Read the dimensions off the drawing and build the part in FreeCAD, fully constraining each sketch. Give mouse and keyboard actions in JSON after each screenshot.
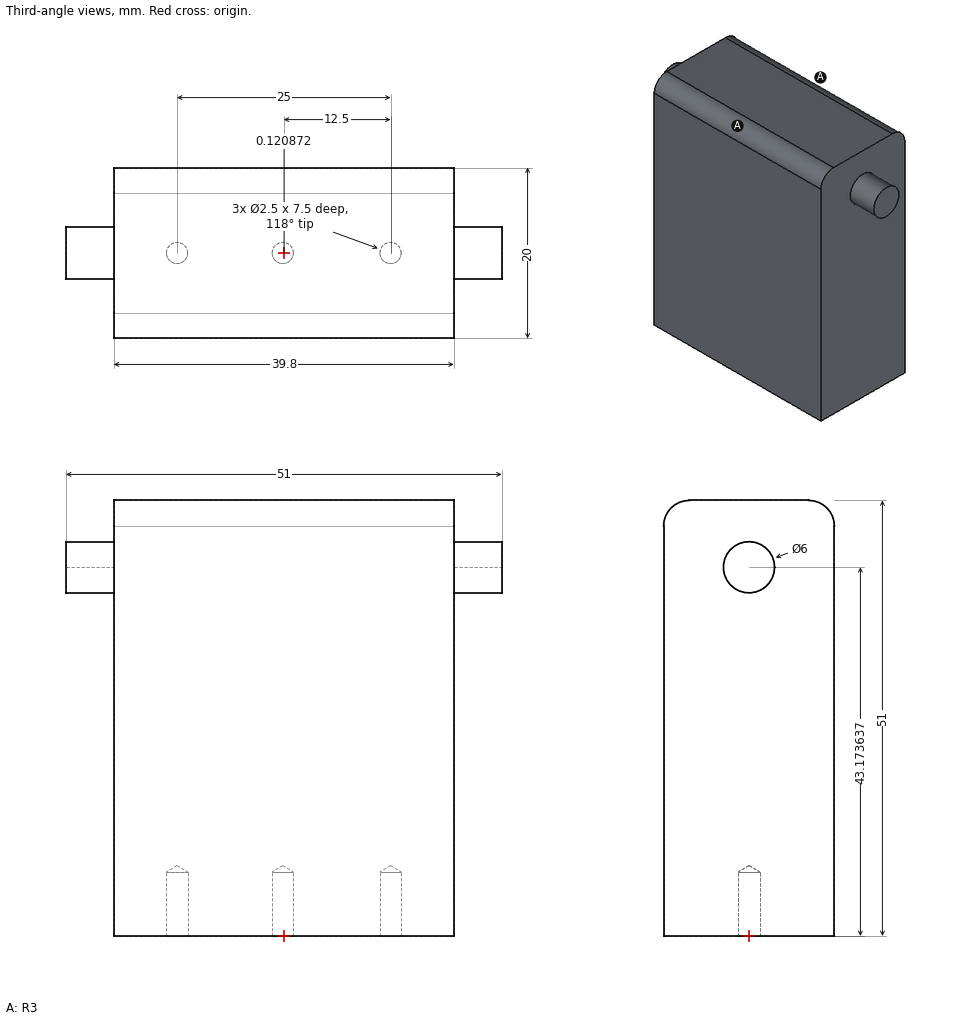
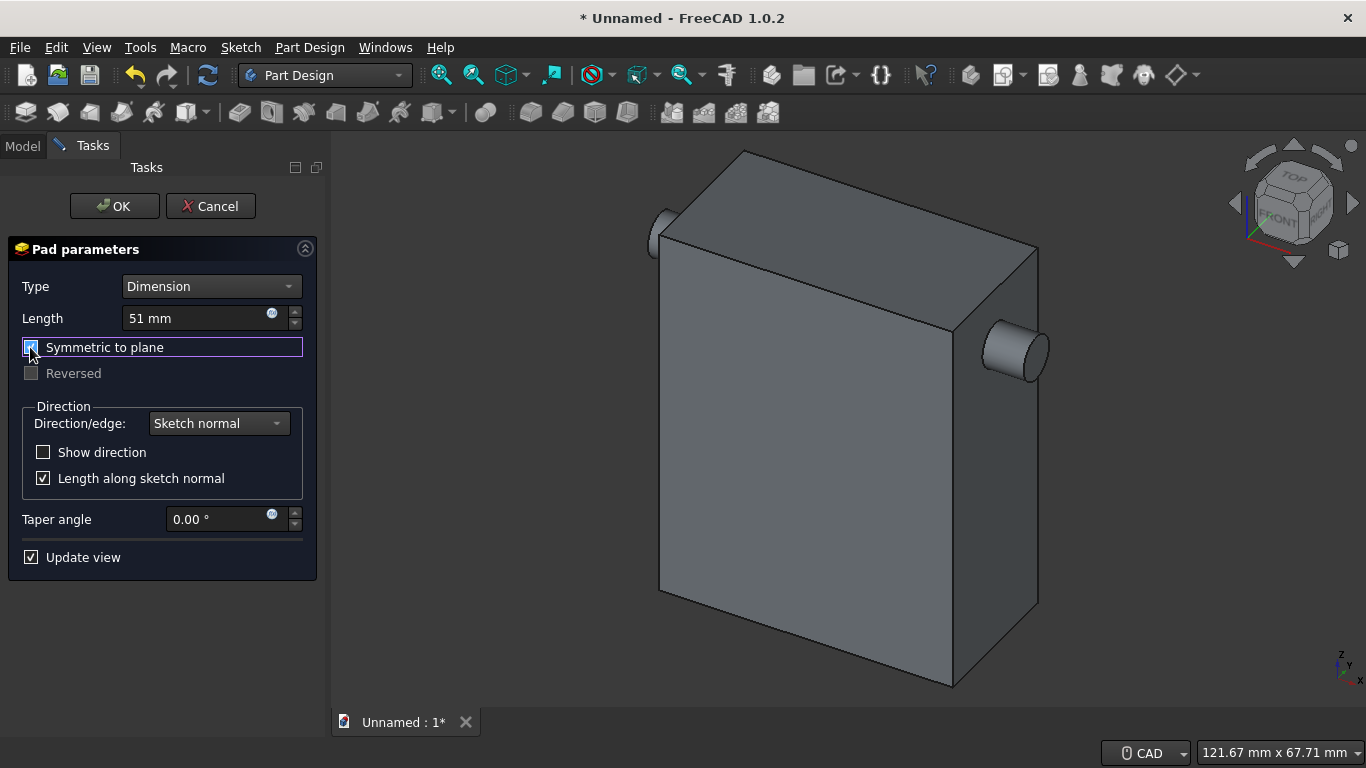
{"action": "left_click", "coordinate": [115, 206]}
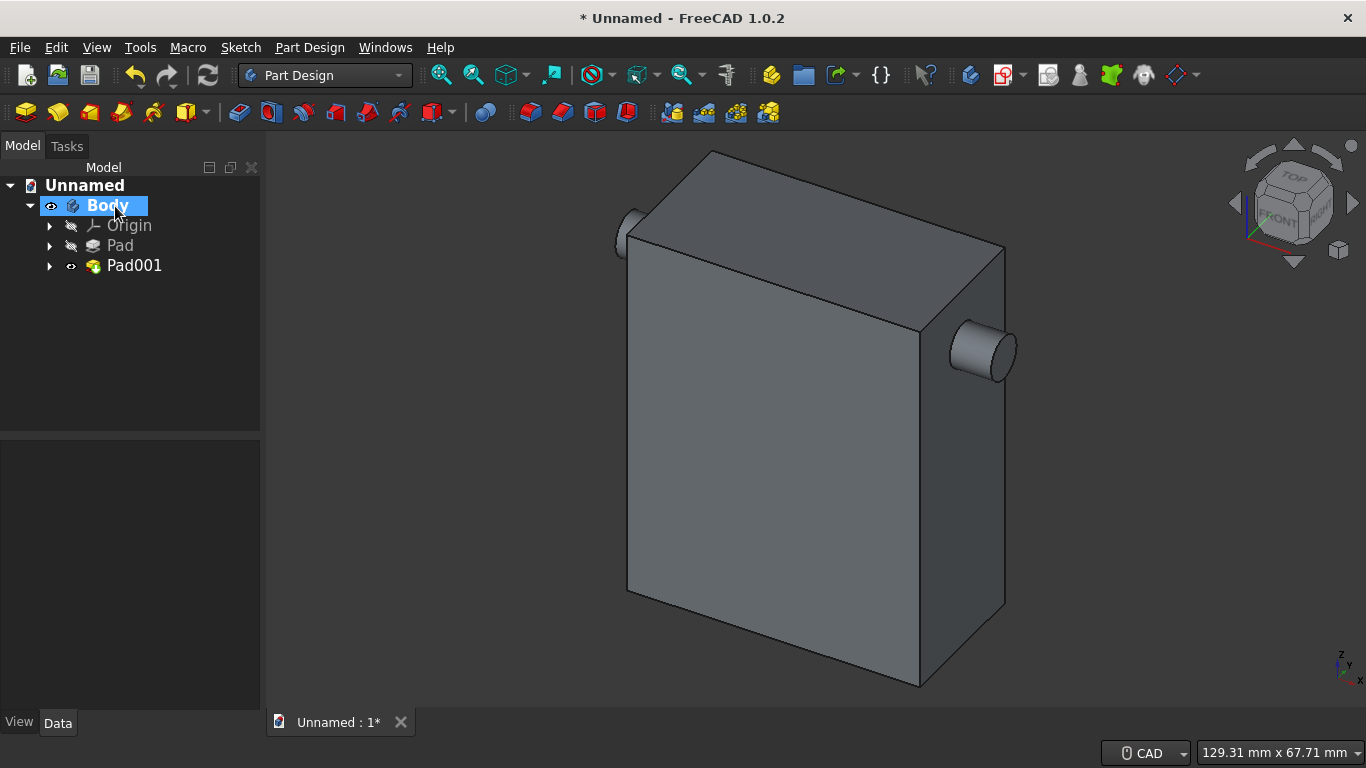
{"action": "key", "text": "5"}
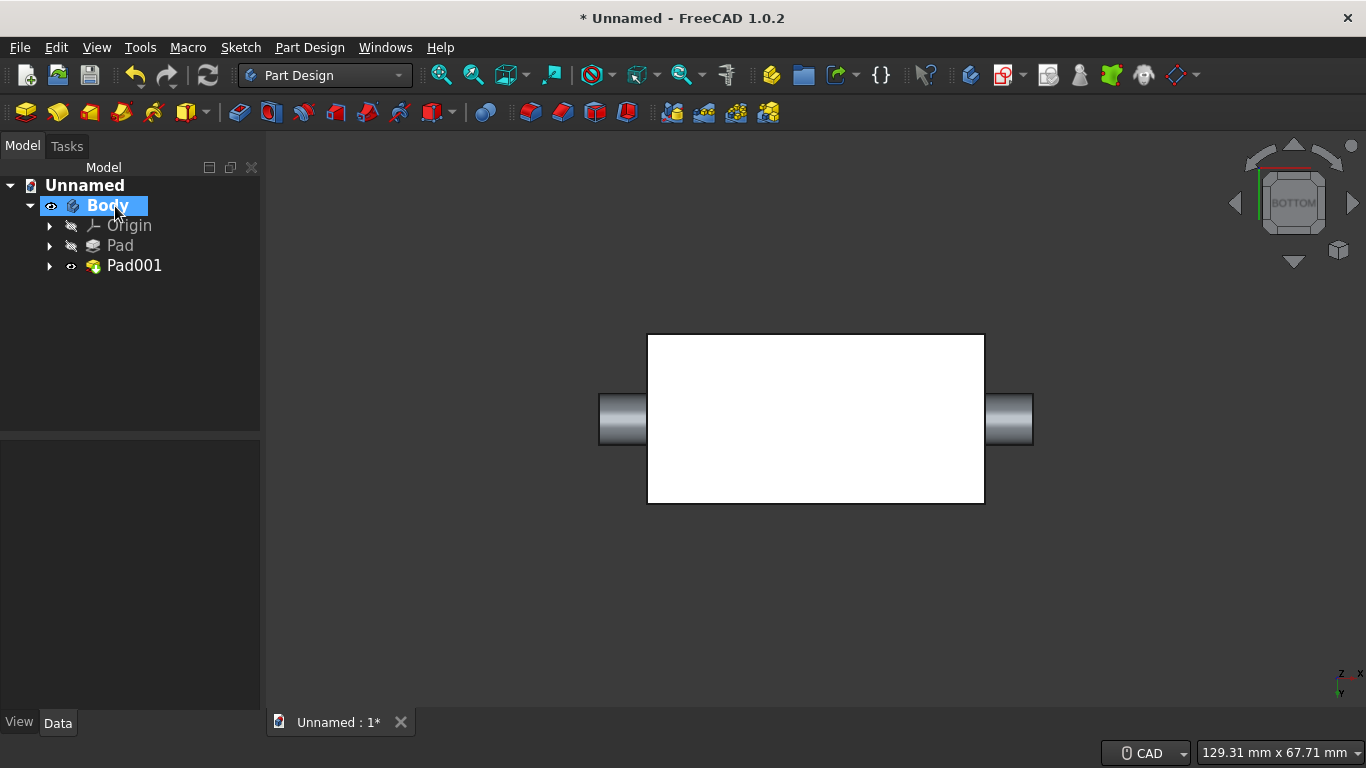
{"action": "key", "text": "v f"}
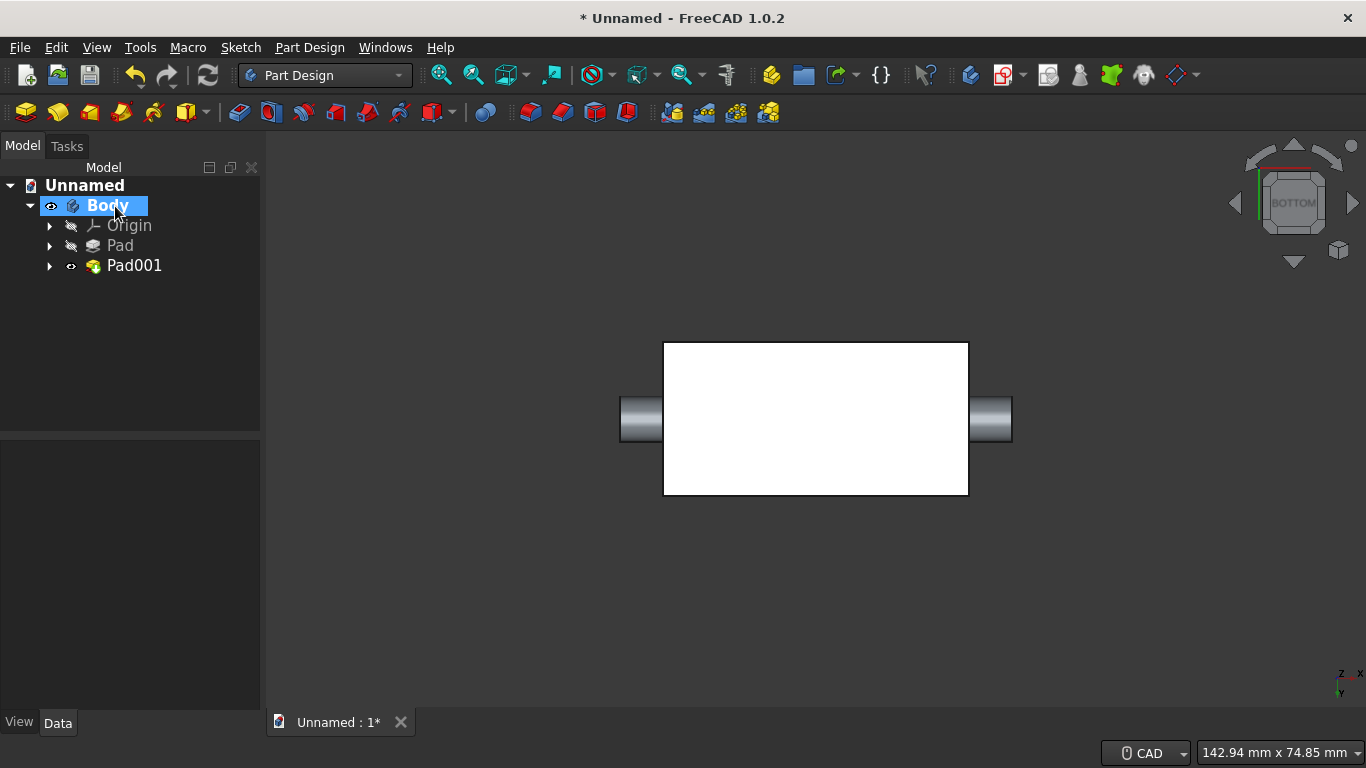
{"action": "left_click", "coordinate": [860, 418]}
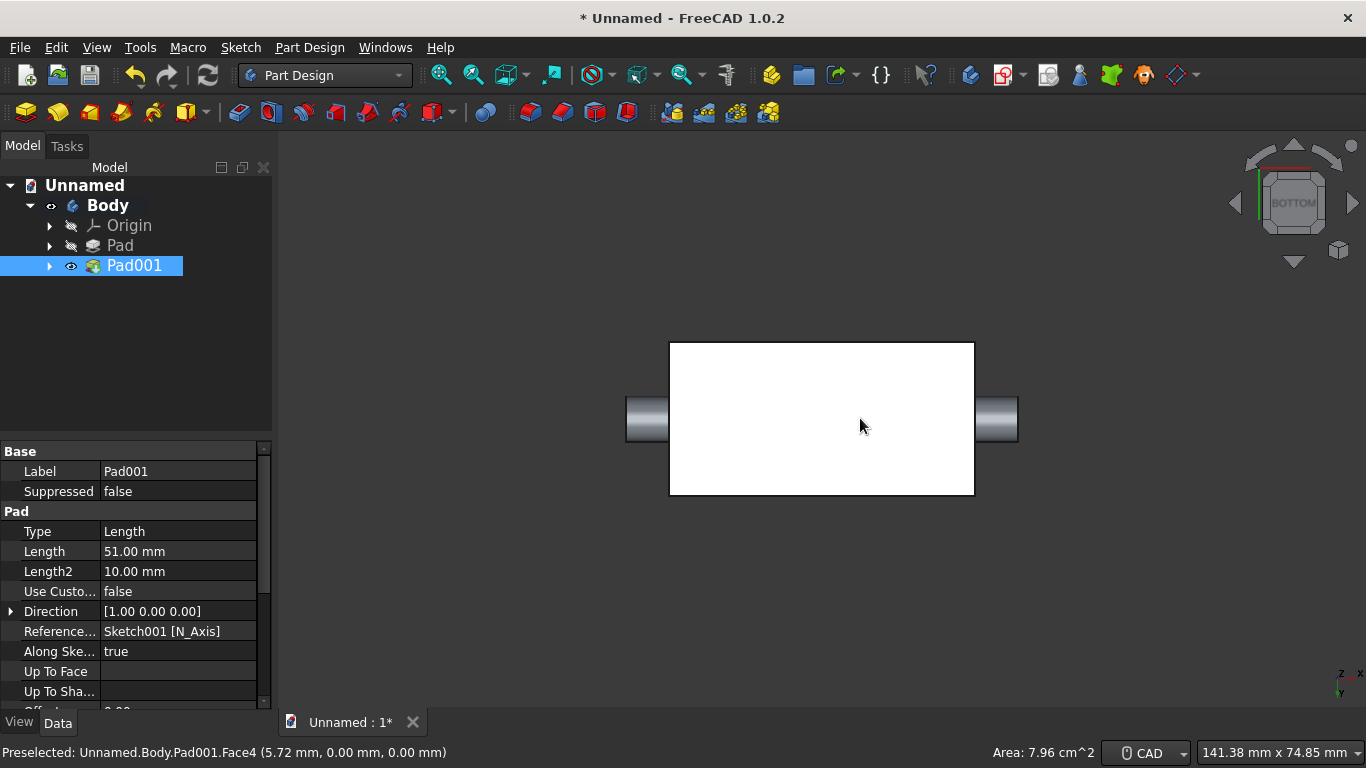
{"action": "left_click", "coordinate": [1004, 76]}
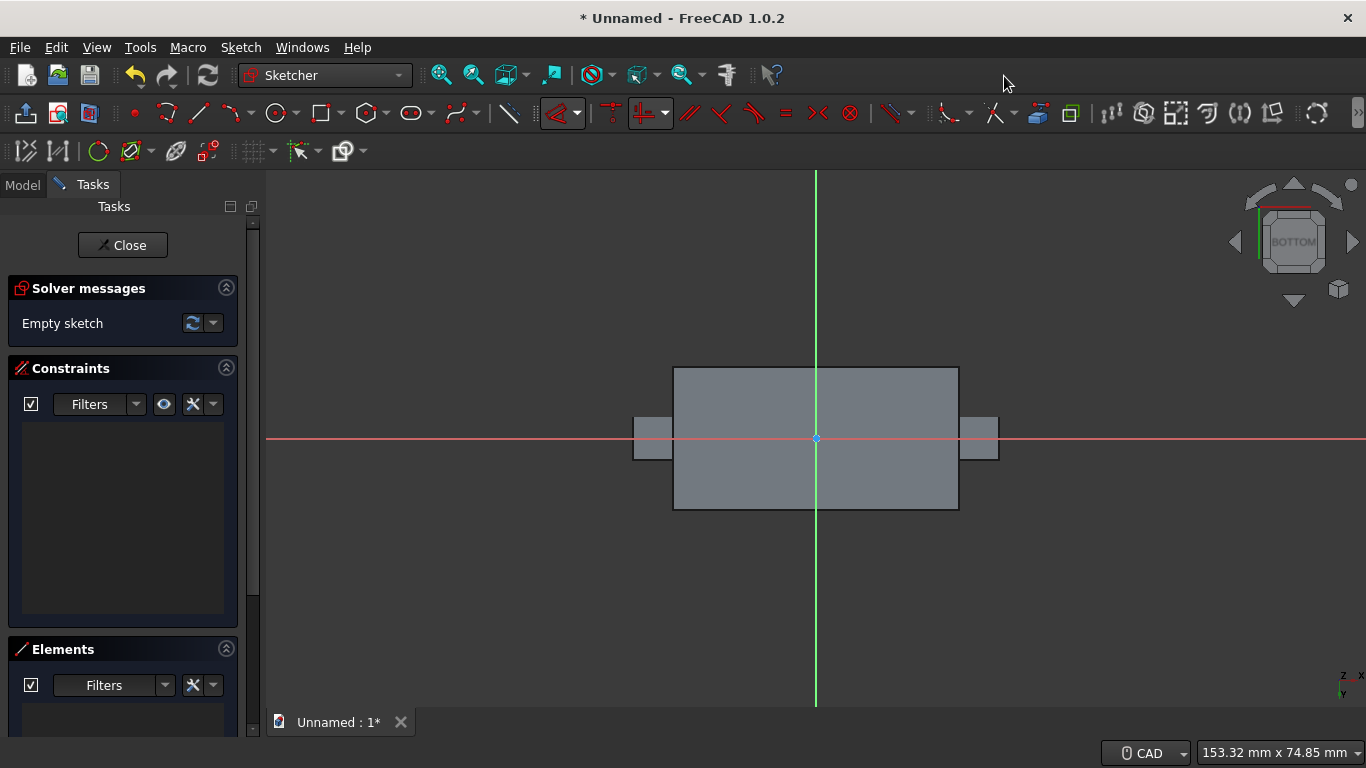
{"action": "scroll", "coordinate": [846, 438], "scroll_direction": "up", "scroll_amount": 6}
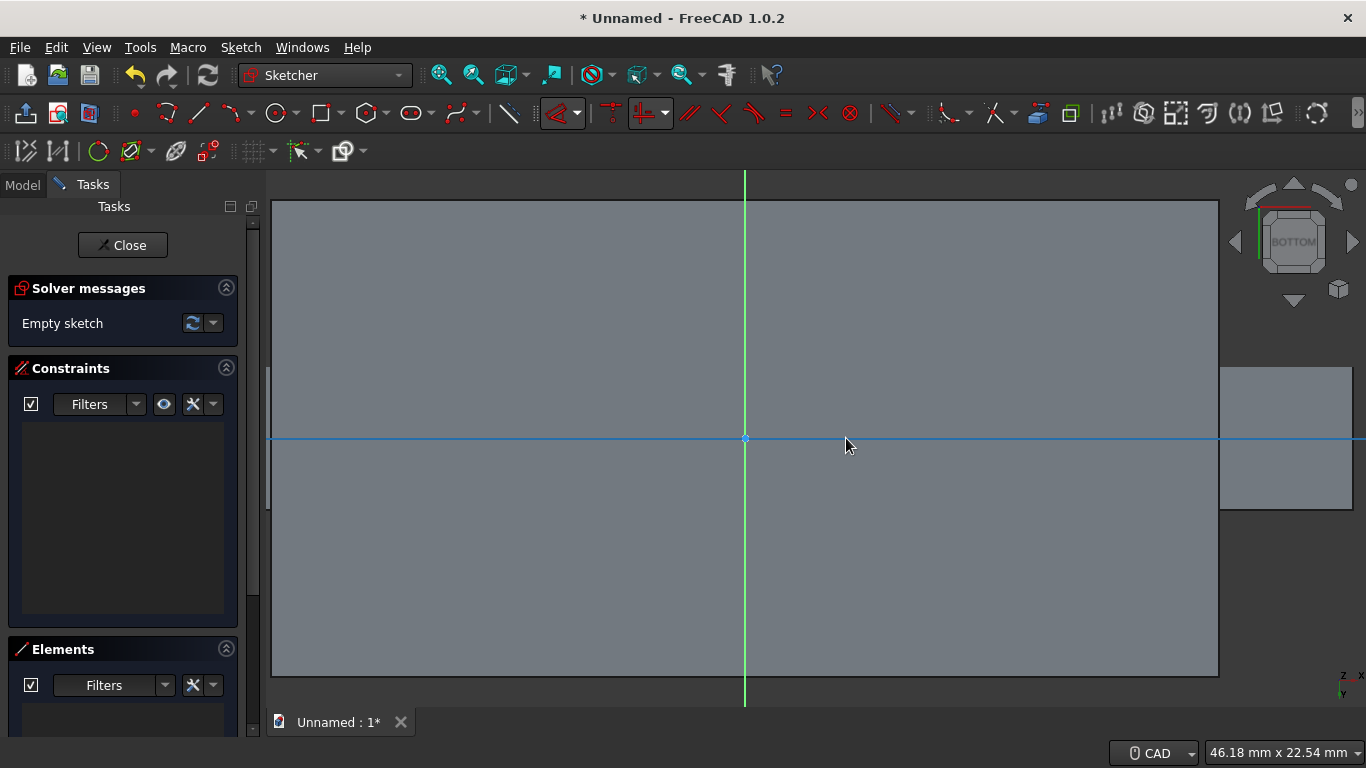
{"action": "key", "text": "g c"}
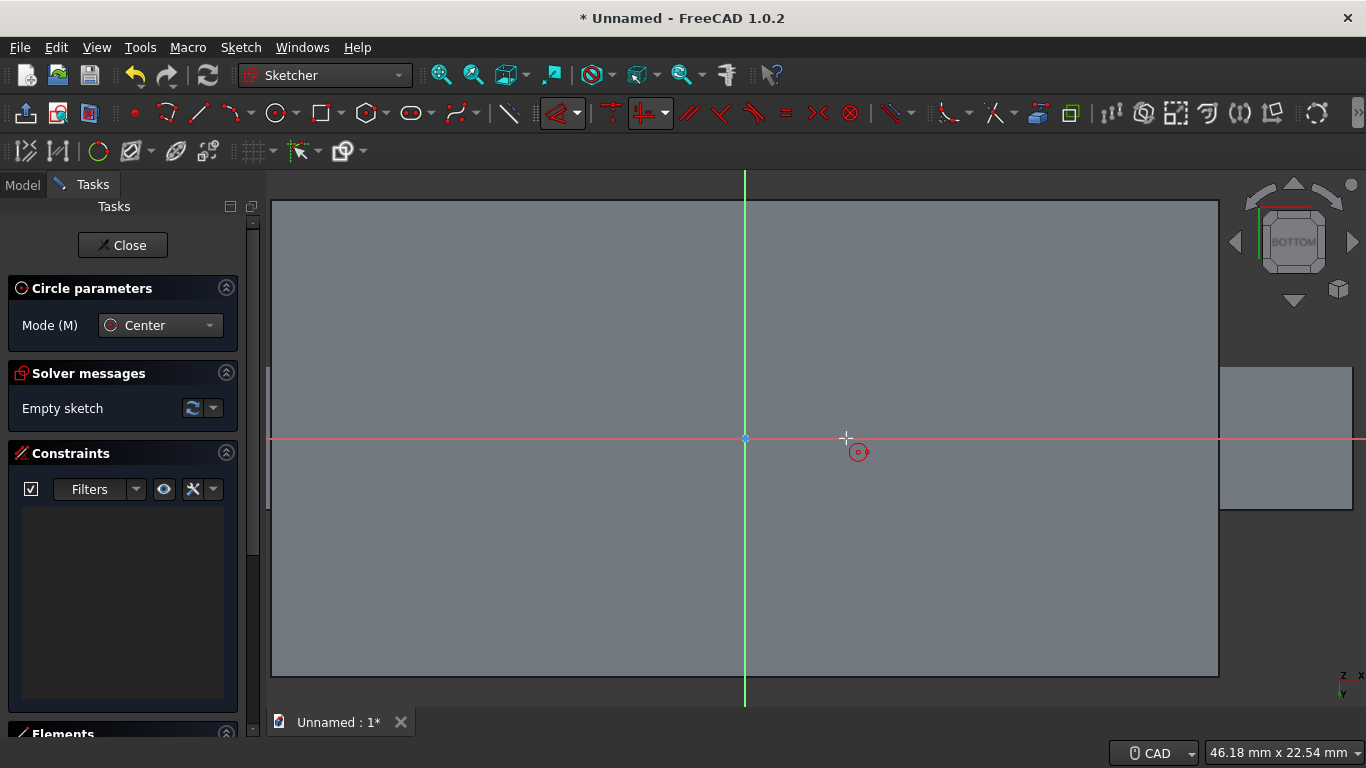
{"action": "left_click", "coordinate": [1043, 438]}
{"action": "left_click", "coordinate": [1064, 417]}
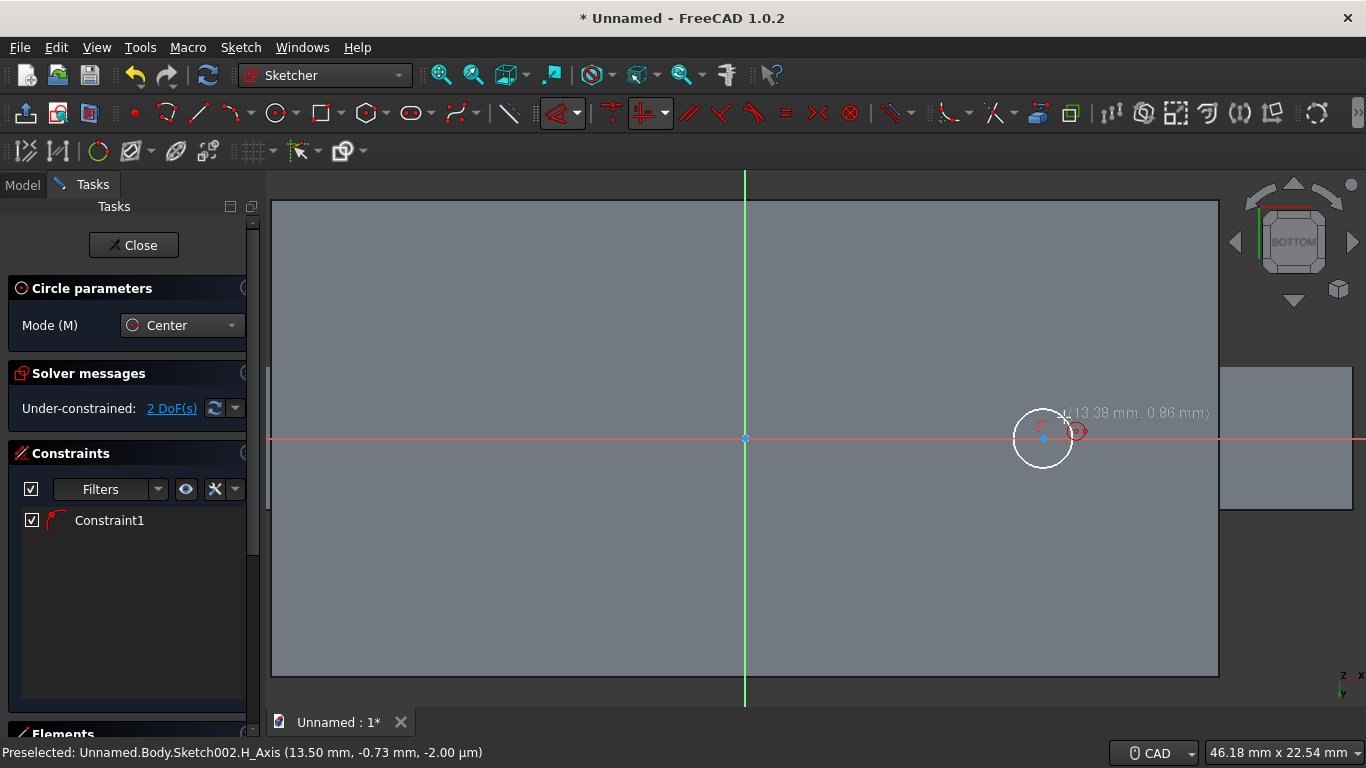
{"action": "left_click", "coordinate": [447, 438]}
{"action": "left_click", "coordinate": [468, 417]}